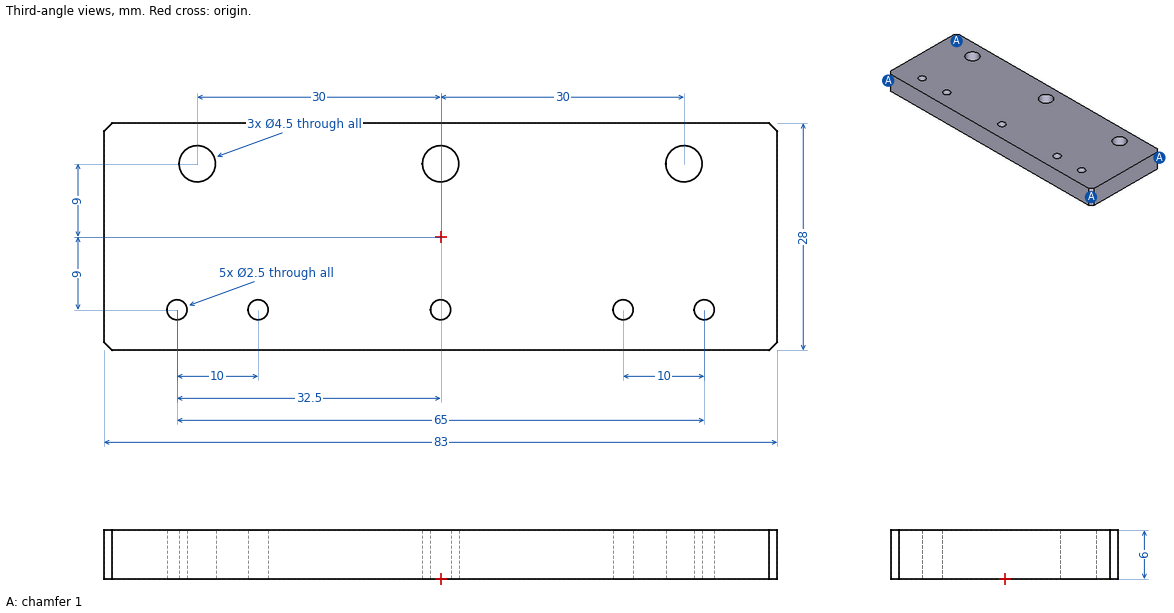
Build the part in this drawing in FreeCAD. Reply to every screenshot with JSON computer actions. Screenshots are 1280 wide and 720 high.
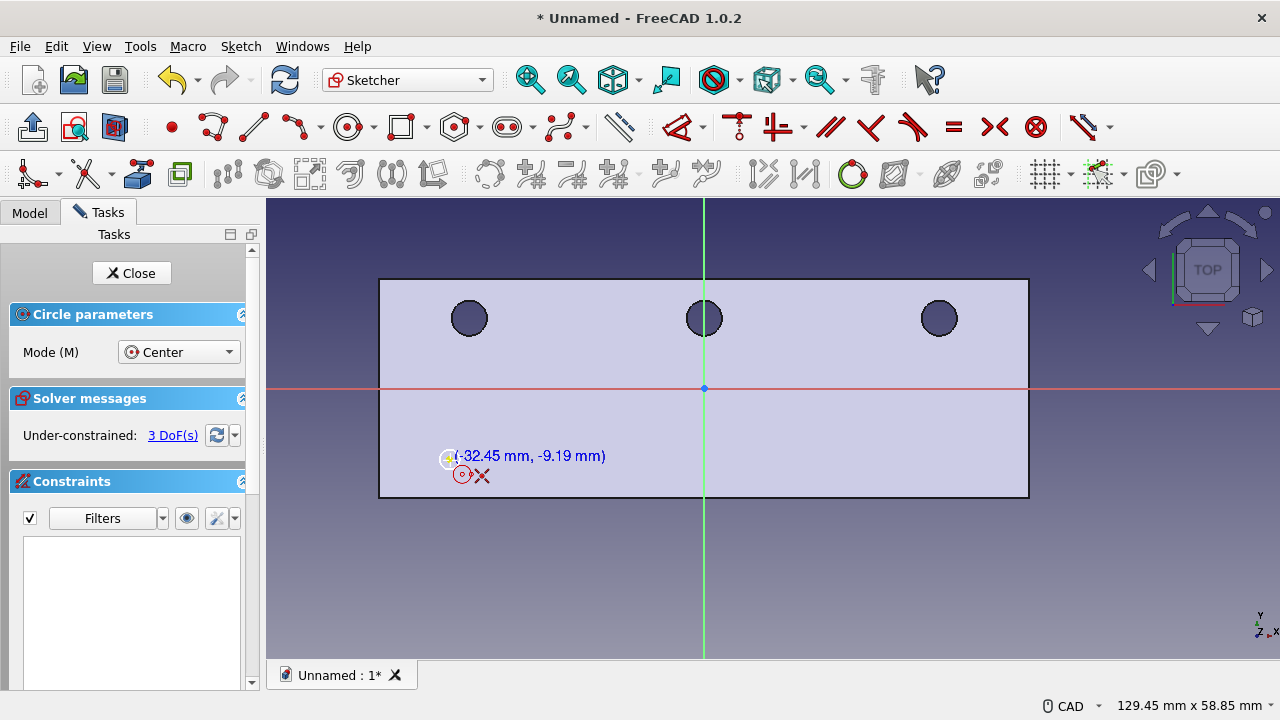
{"action": "scroll", "coordinate": [704, 459], "scroll_direction": "up", "scroll_amount": 5}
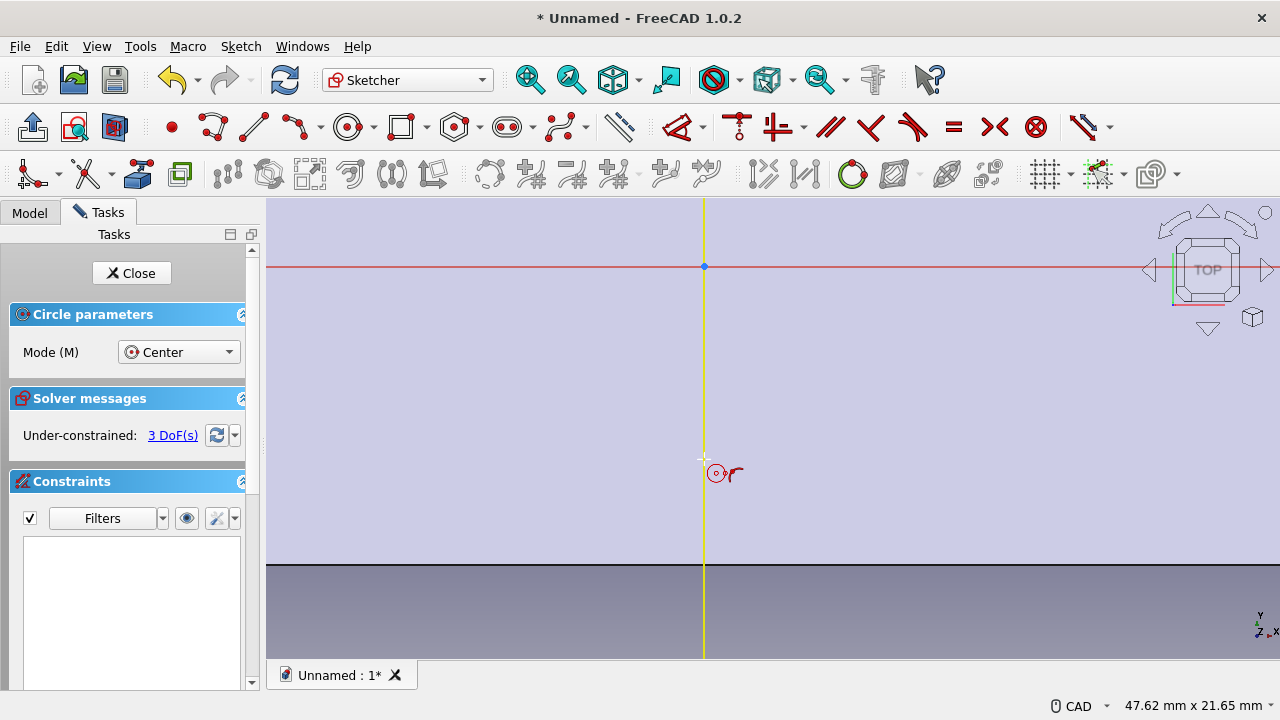
{"action": "left_click", "coordinate": [704, 459]}
{"action": "left_click", "coordinate": [723, 440]}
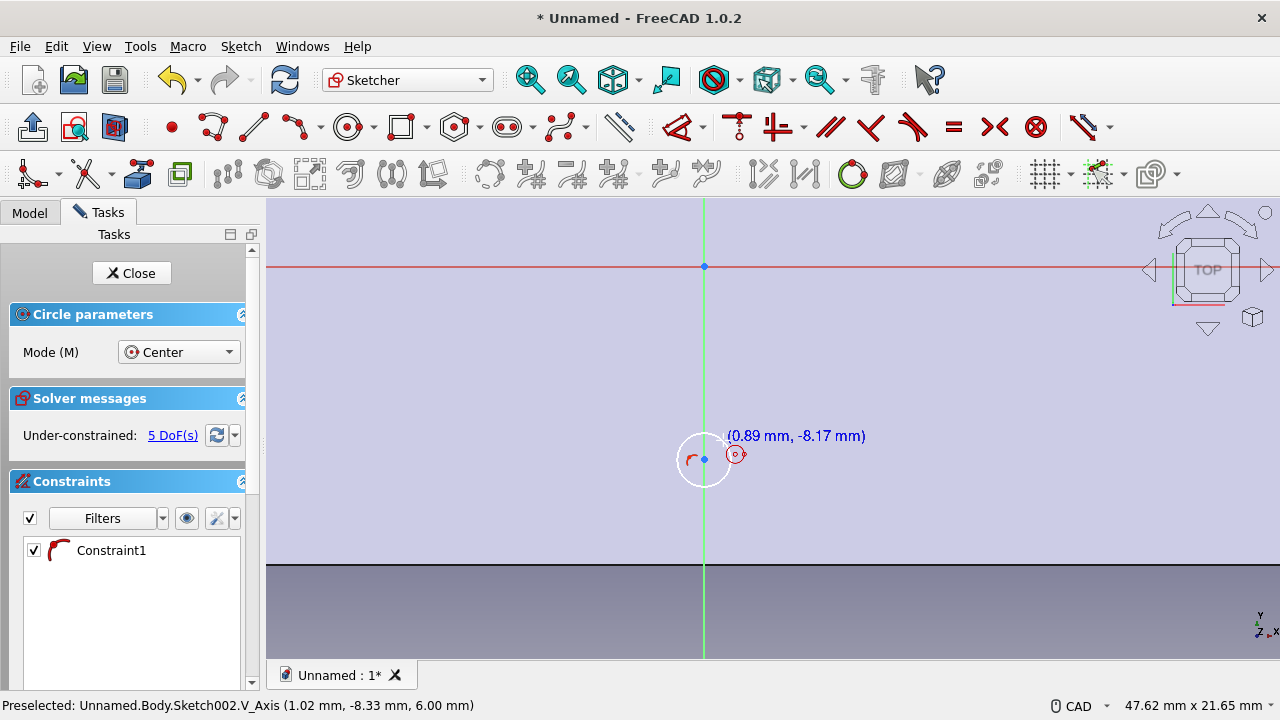
{"action": "scroll", "coordinate": [705, 459], "scroll_direction": "down", "scroll_amount": 5}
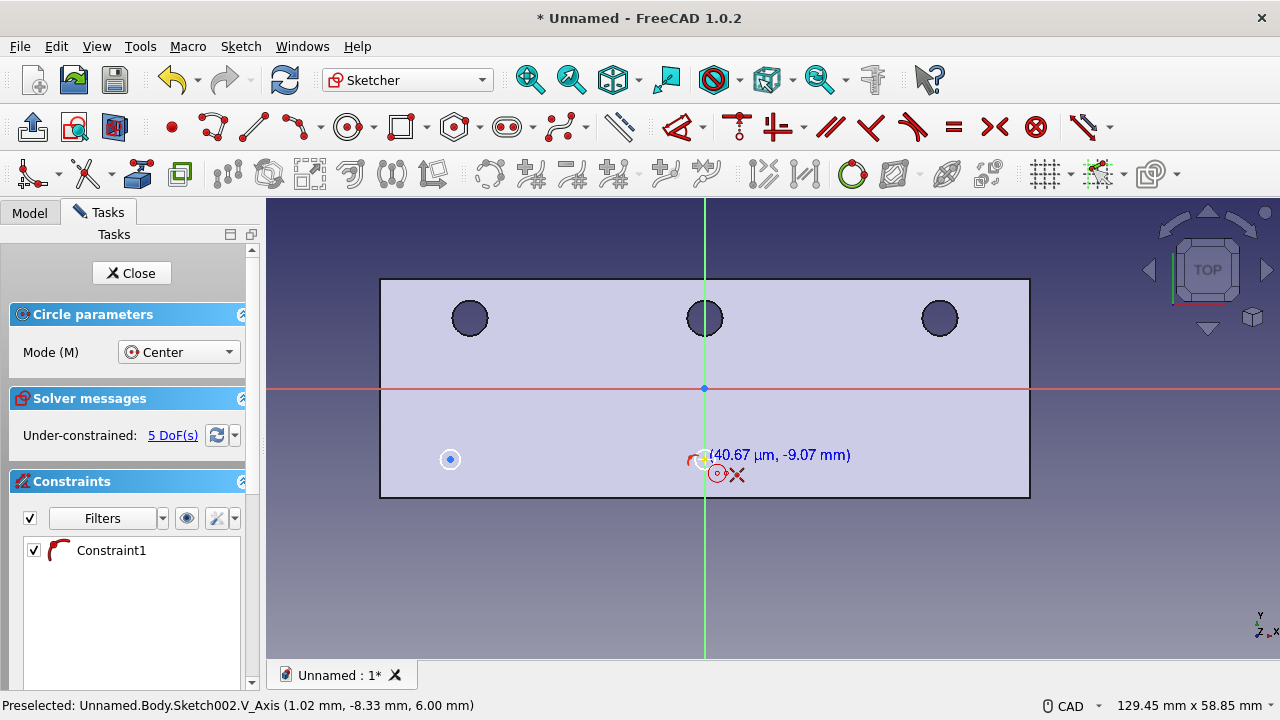
{"action": "scroll", "coordinate": [960, 459], "scroll_direction": "up", "scroll_amount": 5}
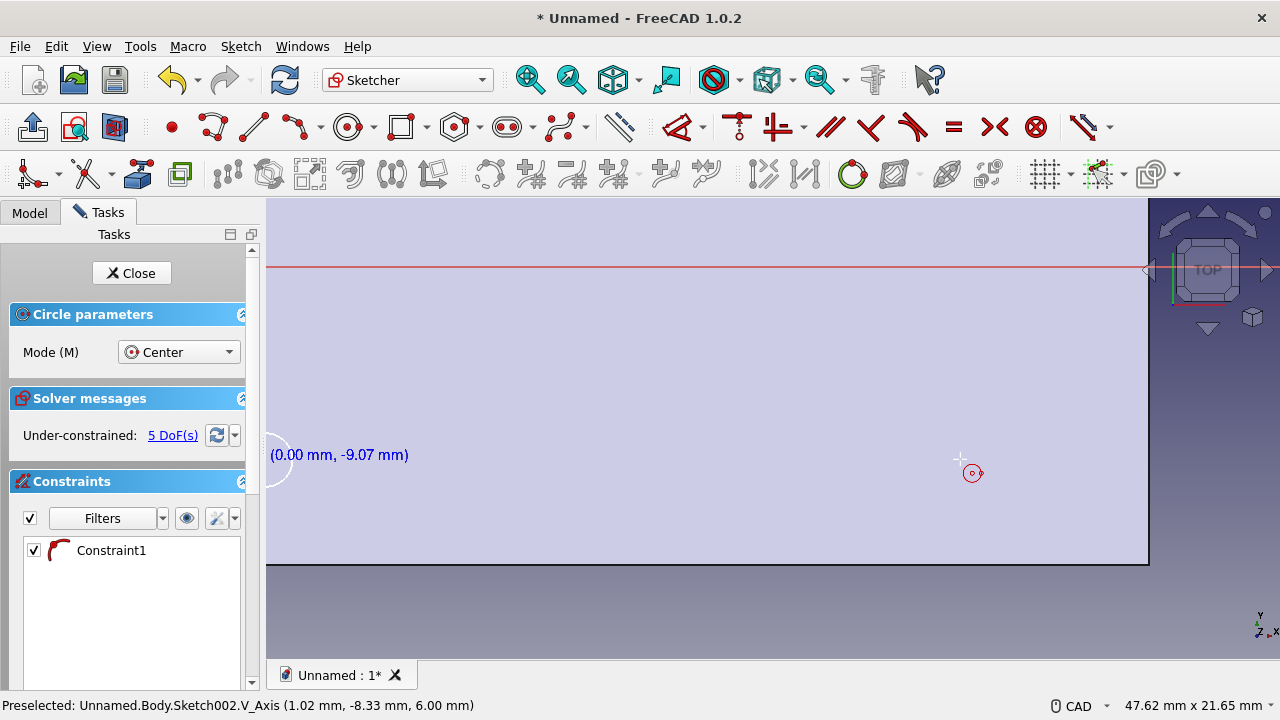
{"action": "left_click", "coordinate": [958, 459]}
{"action": "left_click", "coordinate": [976, 440]}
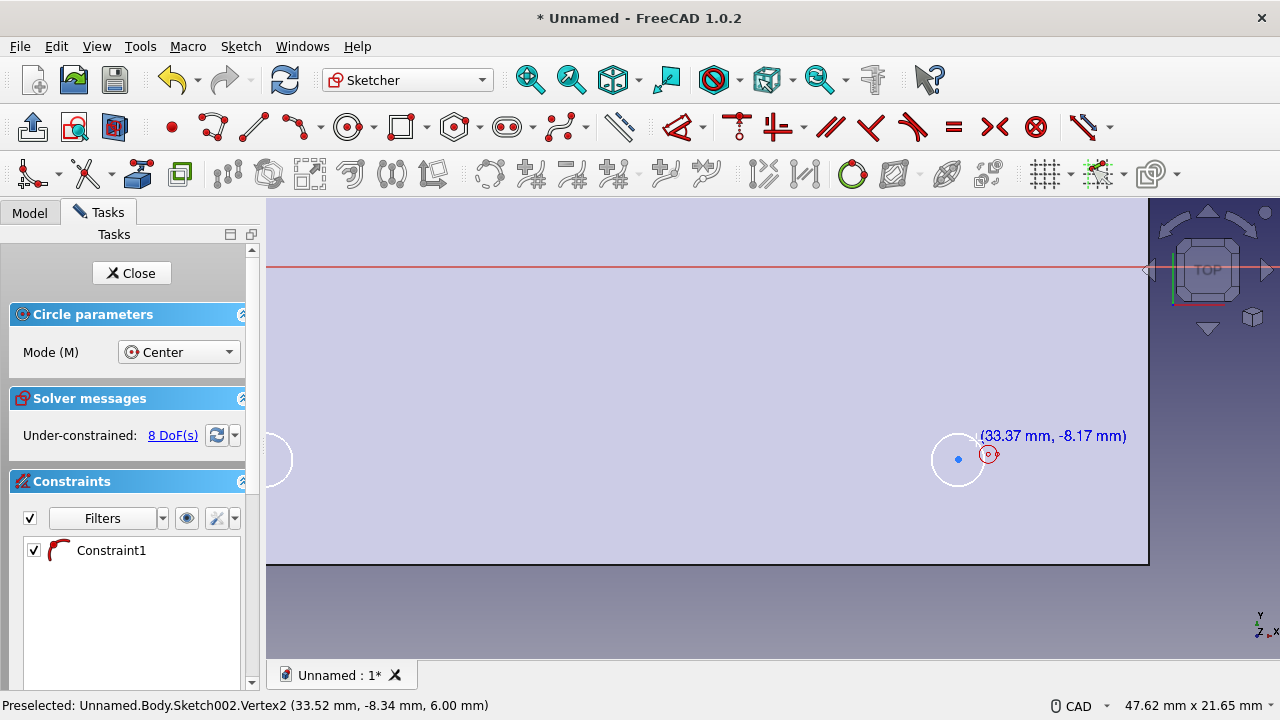
{"action": "left_click", "coordinate": [745, 459]}
{"action": "left_click", "coordinate": [763, 440]}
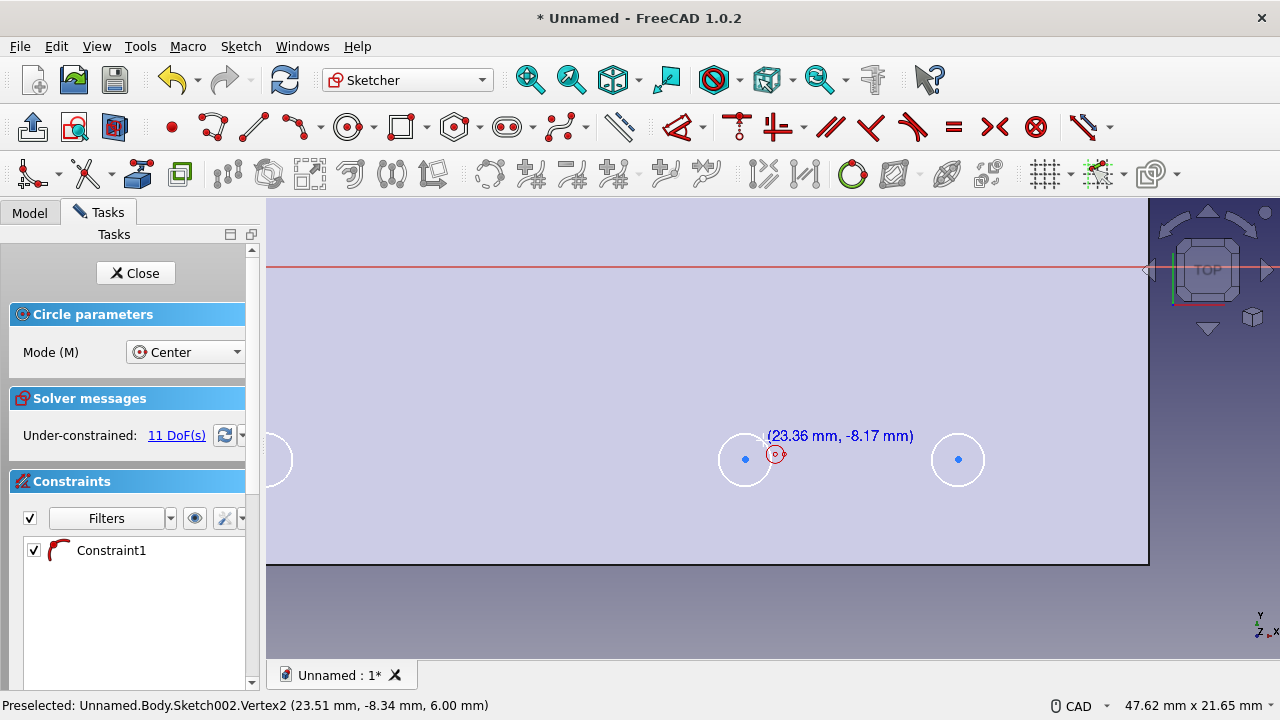
{"action": "scroll", "coordinate": [960, 459], "scroll_direction": "down", "scroll_amount": 5}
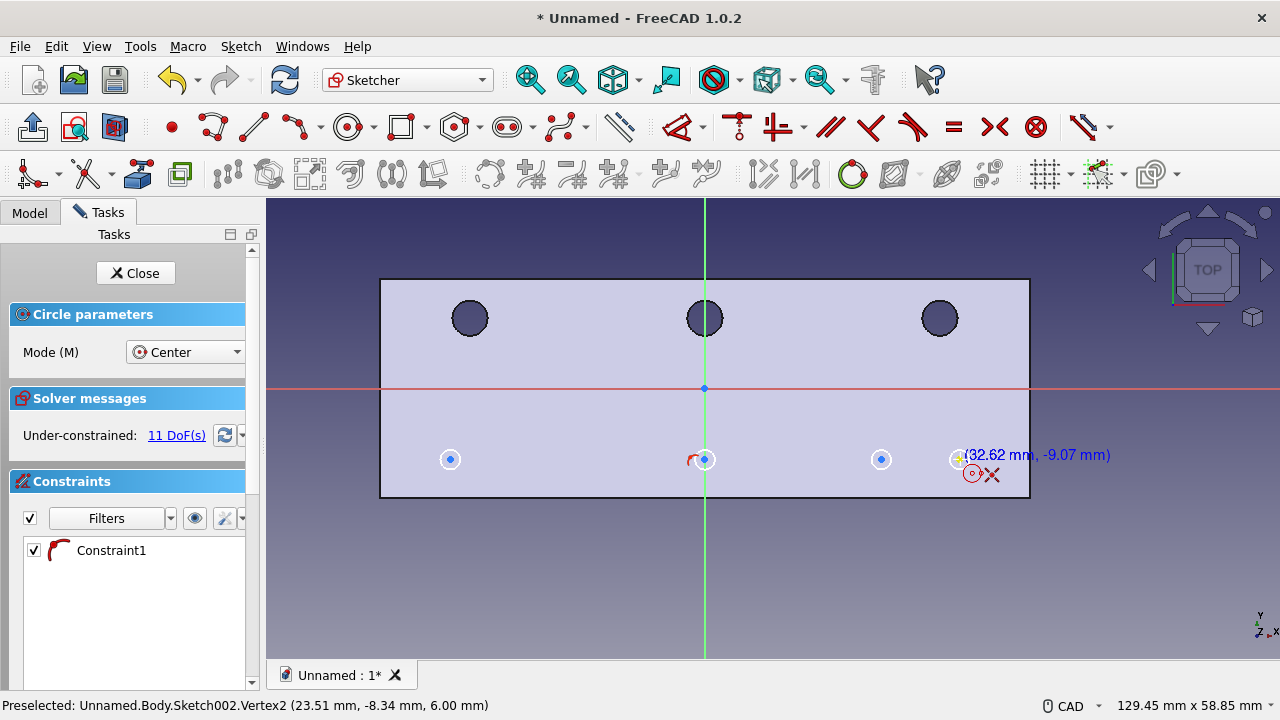
{"action": "scroll", "coordinate": [529, 459], "scroll_direction": "up", "scroll_amount": 5}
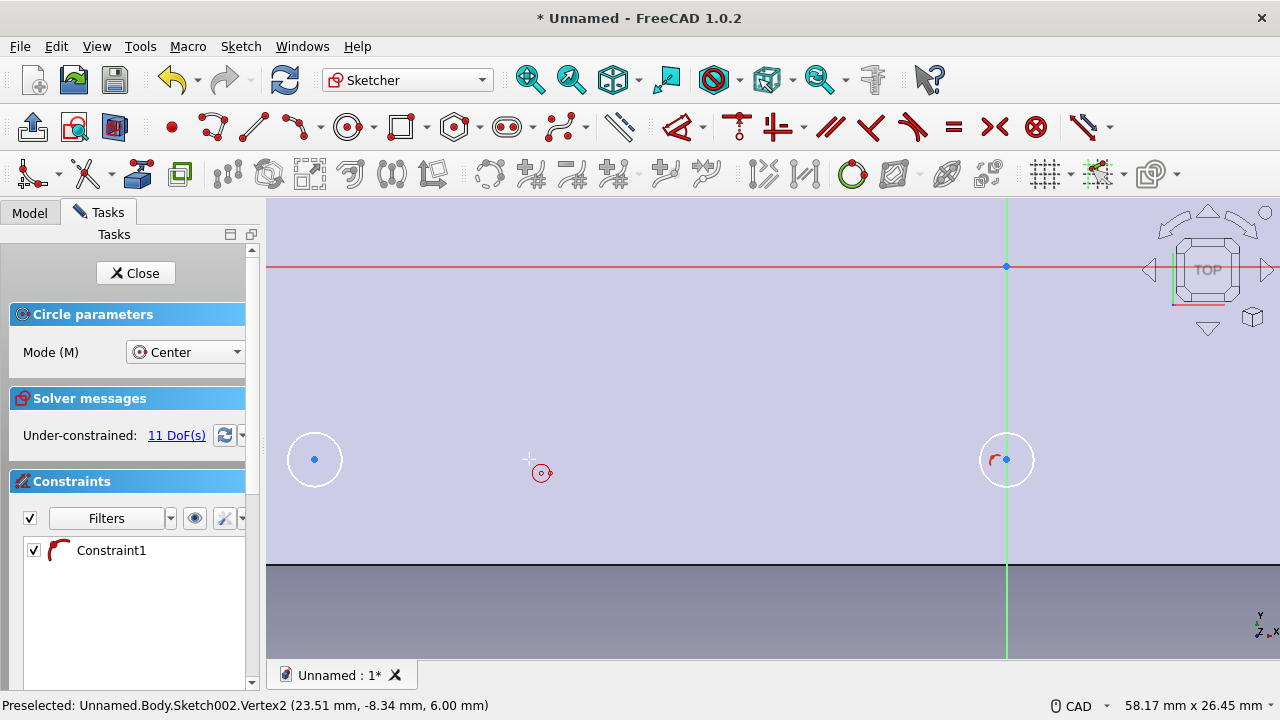
{"action": "left_click", "coordinate": [528, 459]}
{"action": "left_click", "coordinate": [547, 440]}
{"action": "key", "text": "Escape"}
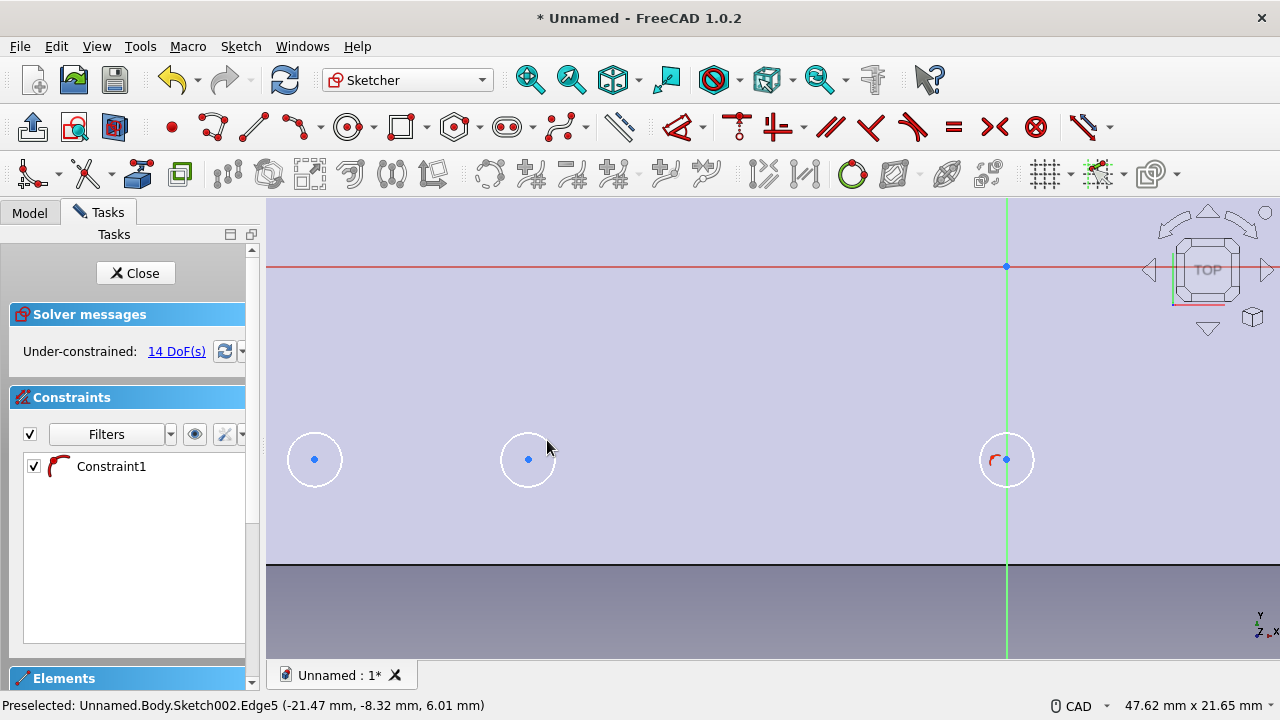
{"action": "left_click", "coordinate": [334, 441]}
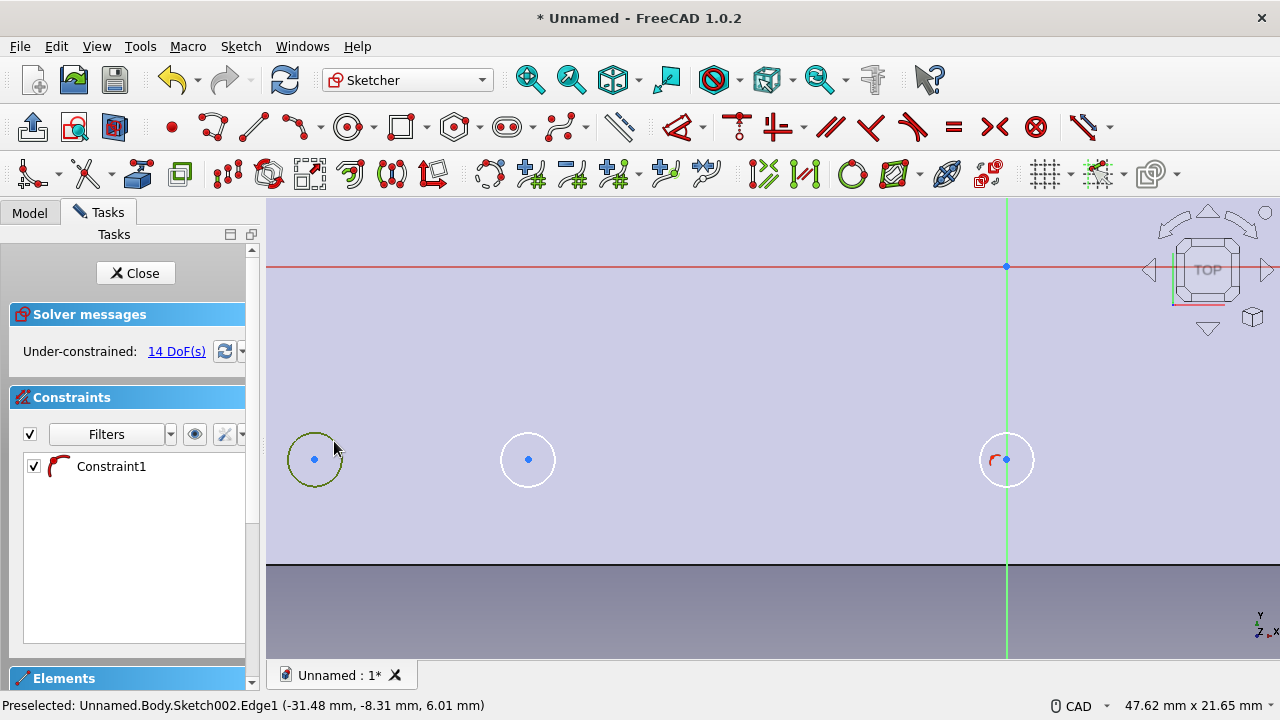
{"action": "left_click", "coordinate": [1026, 441]}